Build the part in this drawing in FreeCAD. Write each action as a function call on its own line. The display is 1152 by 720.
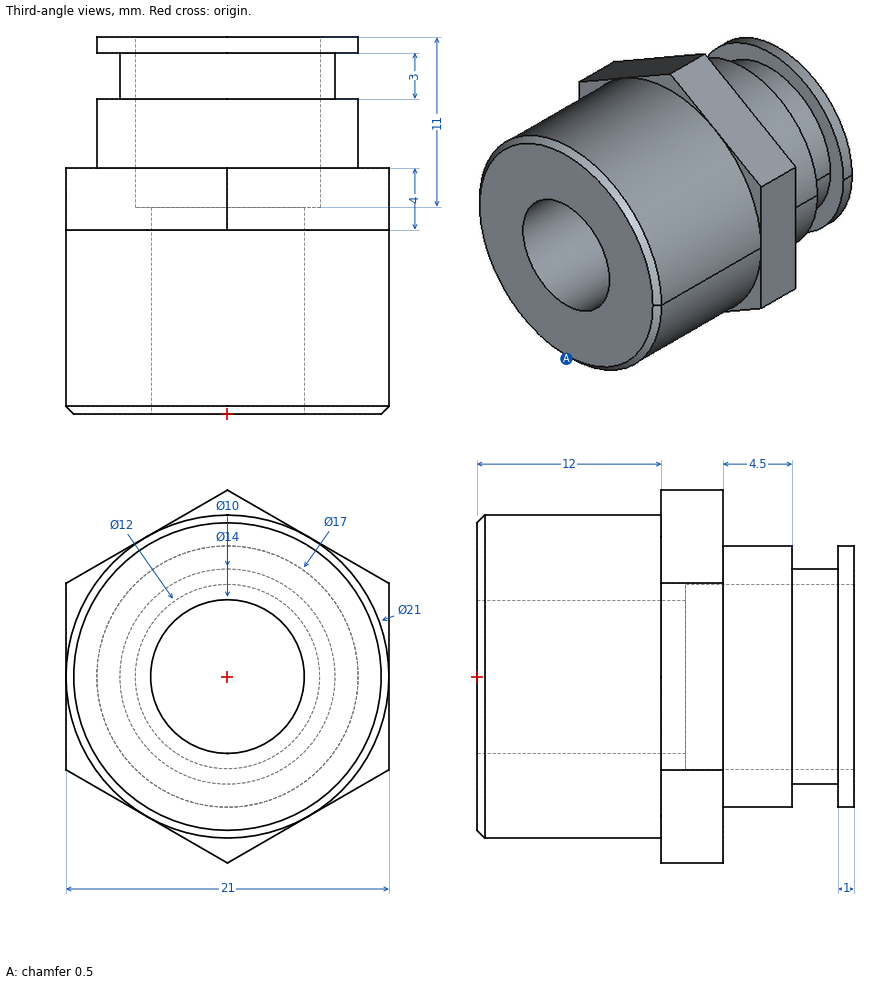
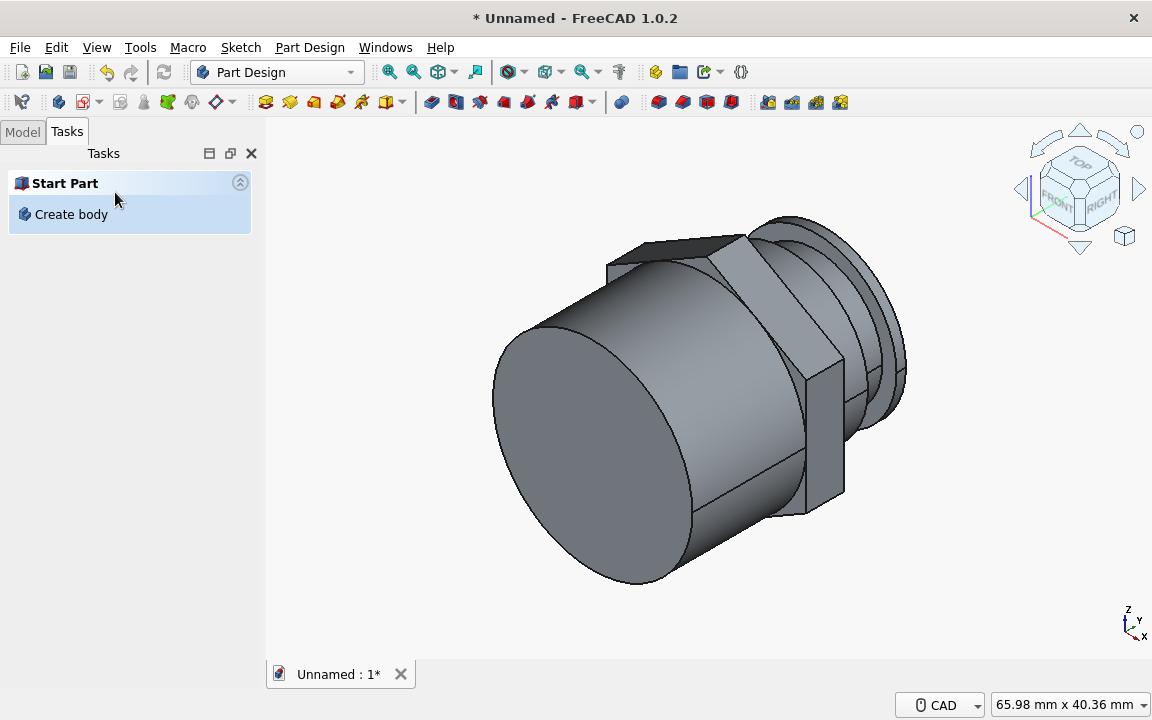
click(512, 340)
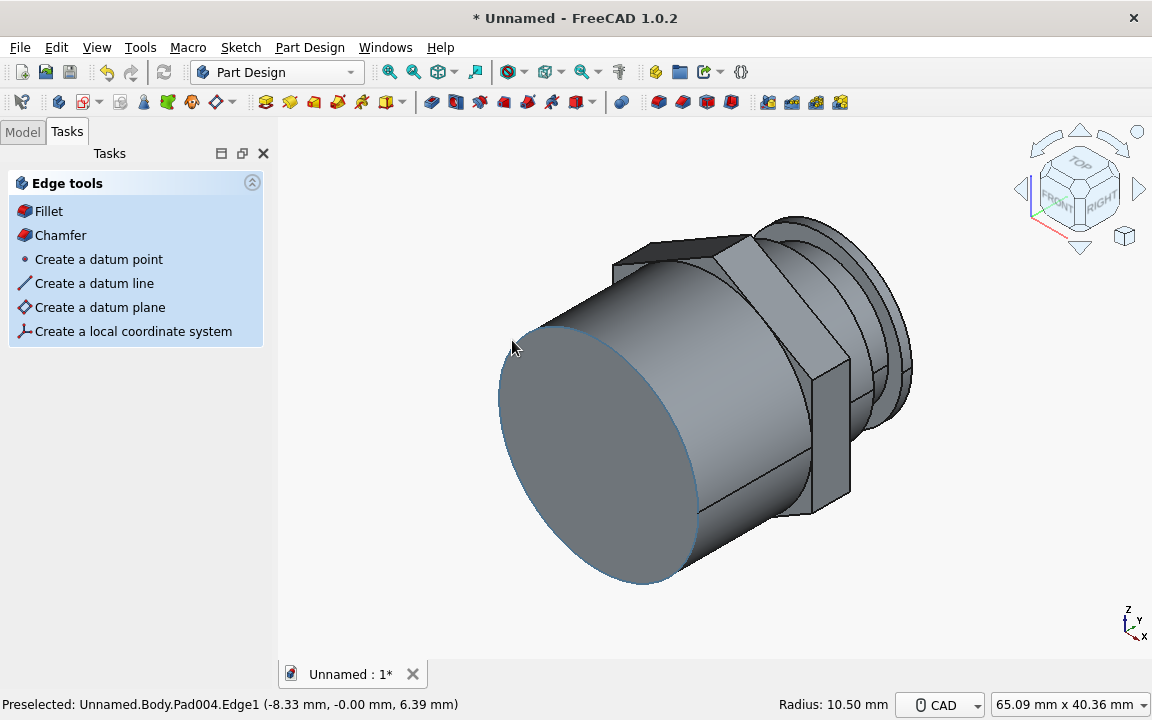
click(684, 102)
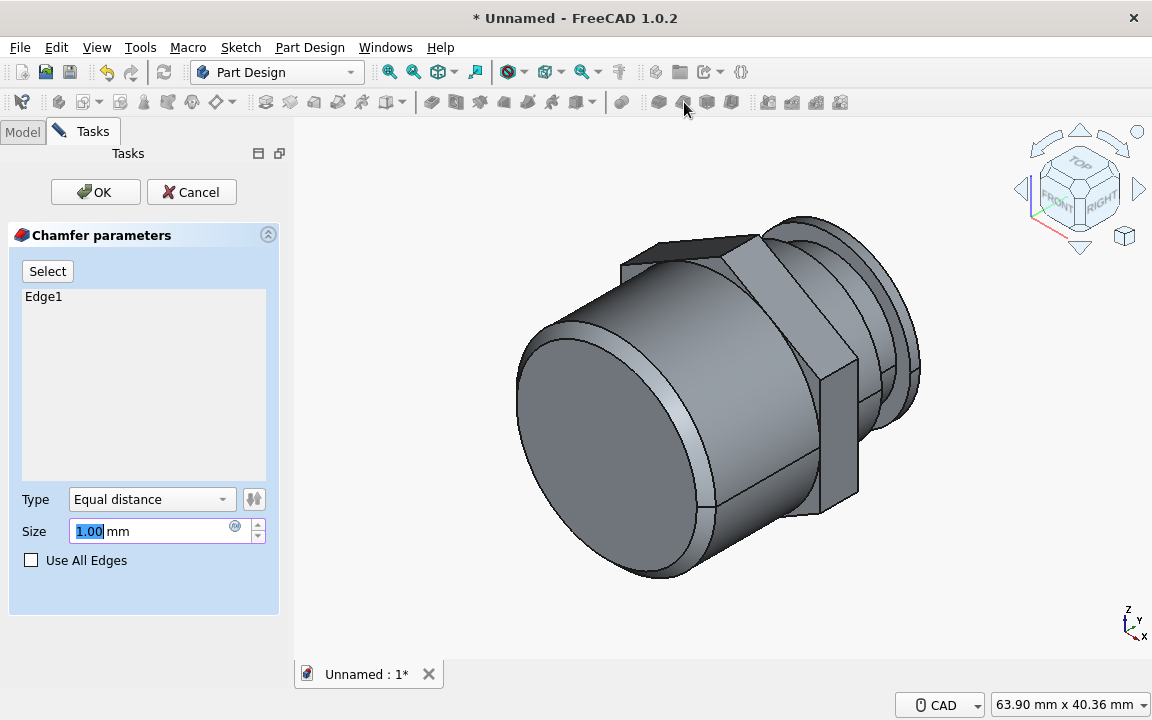
text(0.5)
key(Tab)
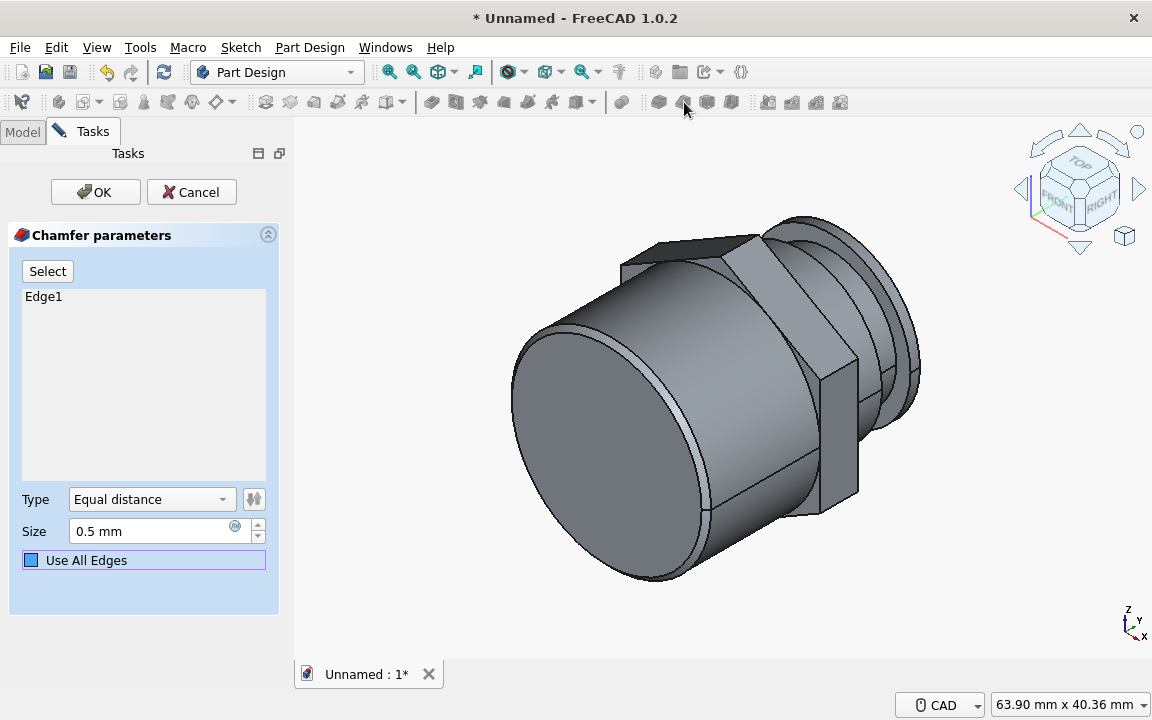
click(96, 192)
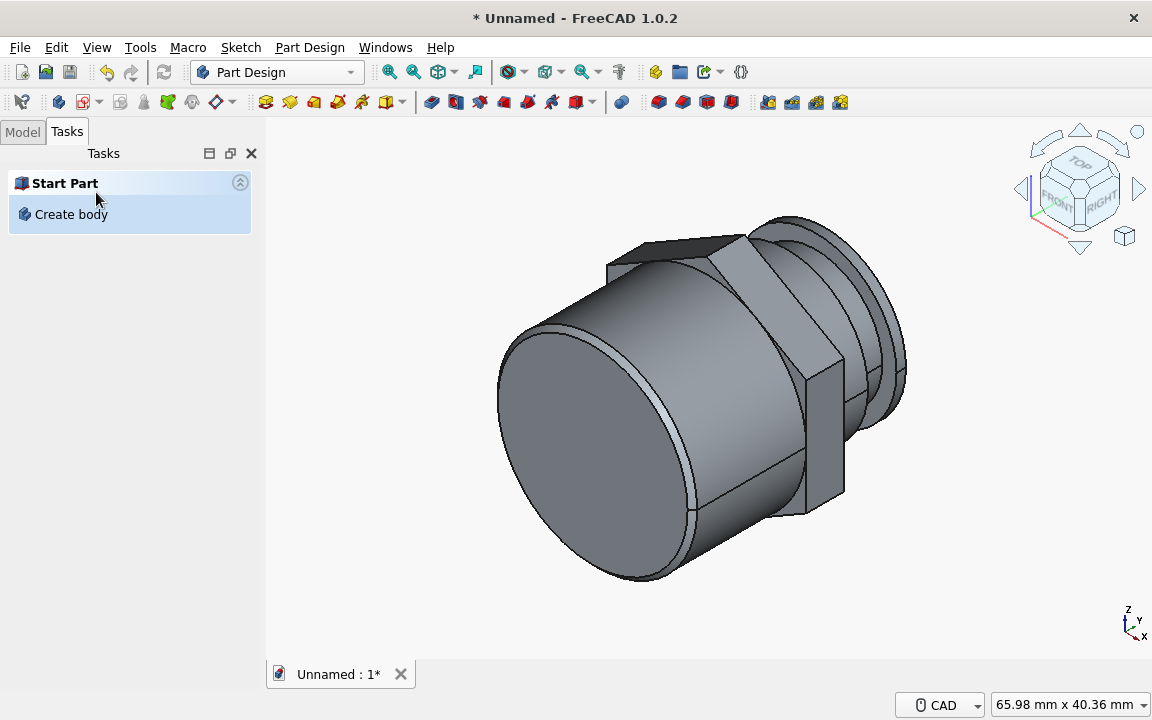
key(4)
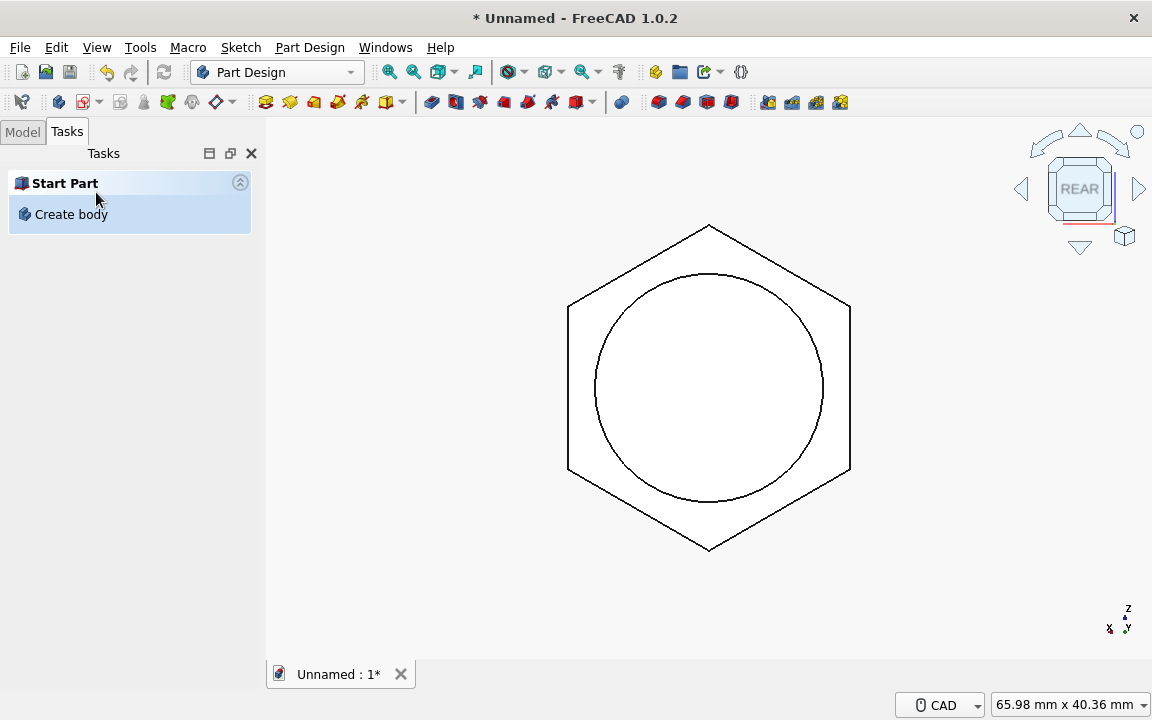
click(709, 387)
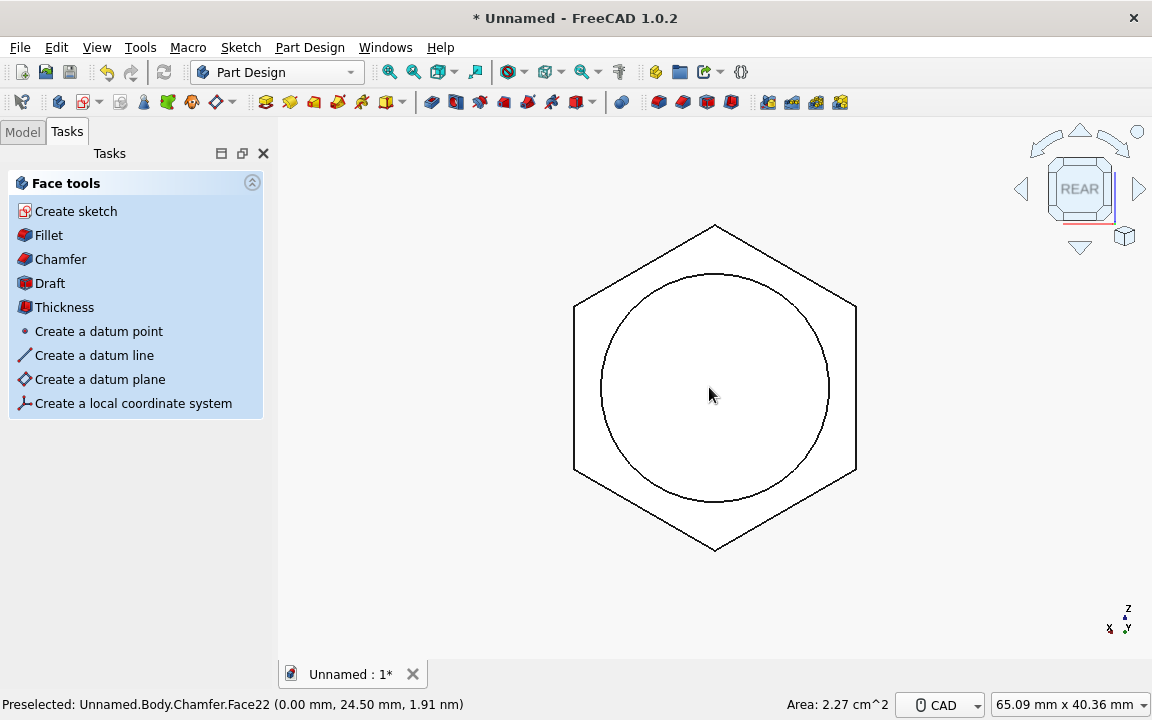
click(84, 102)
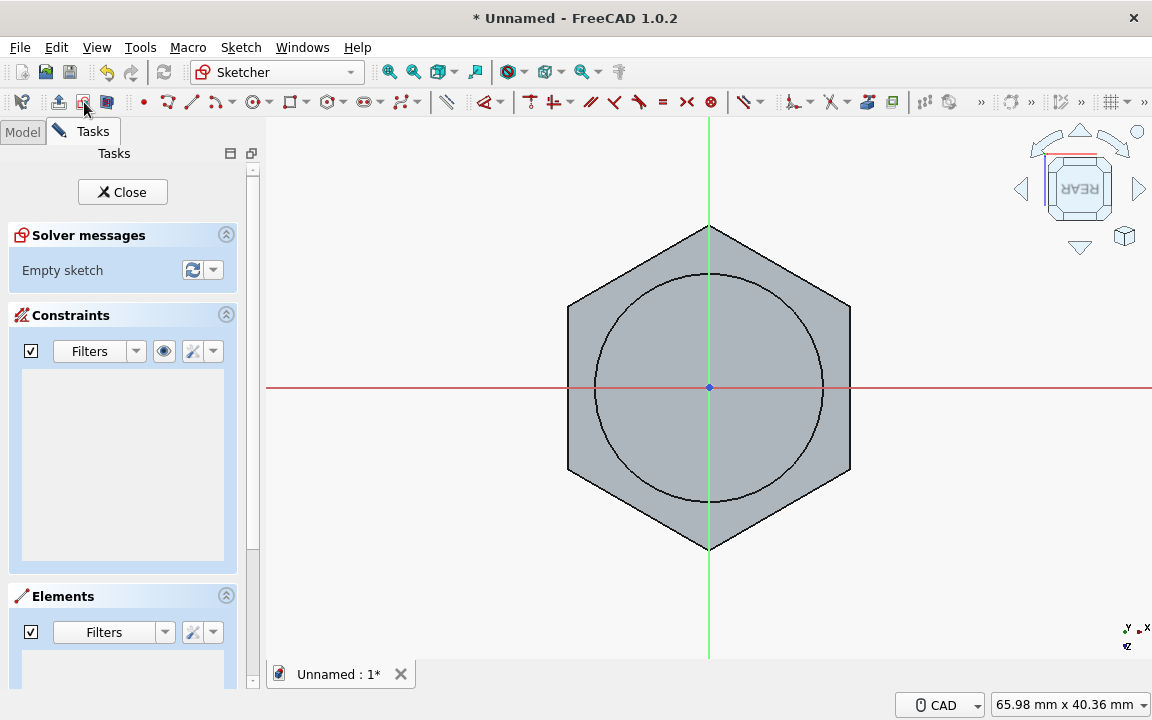
scroll(765, 388, up, 4)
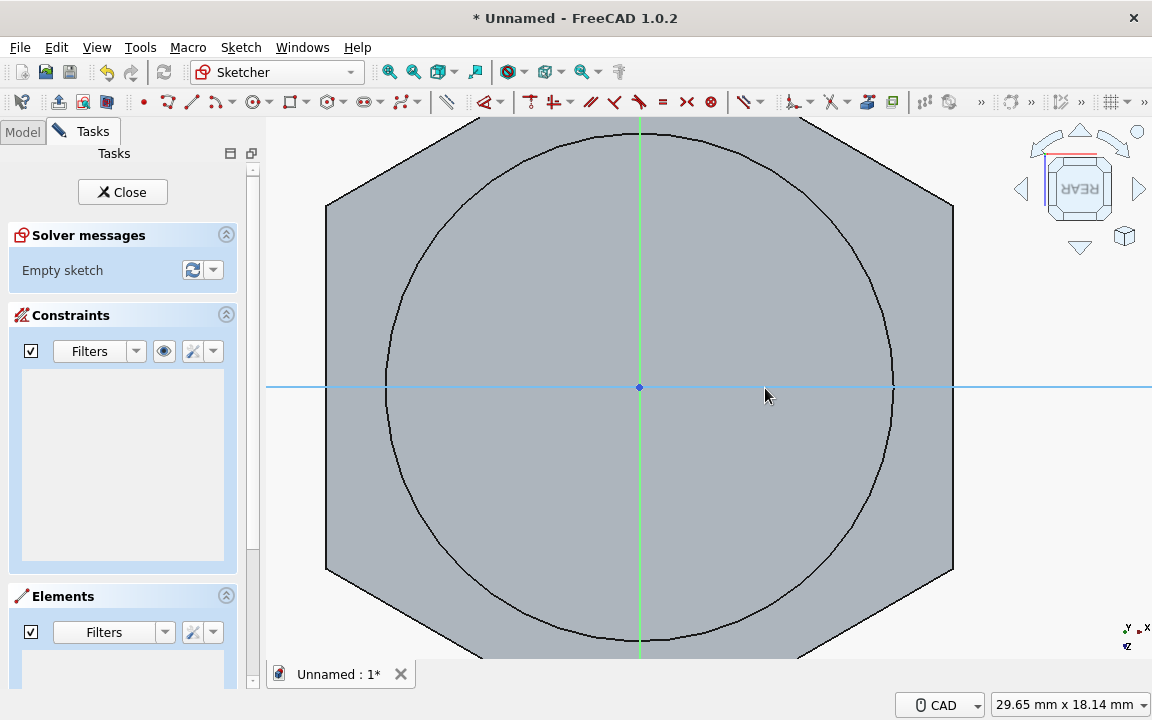
key(g)
key(c)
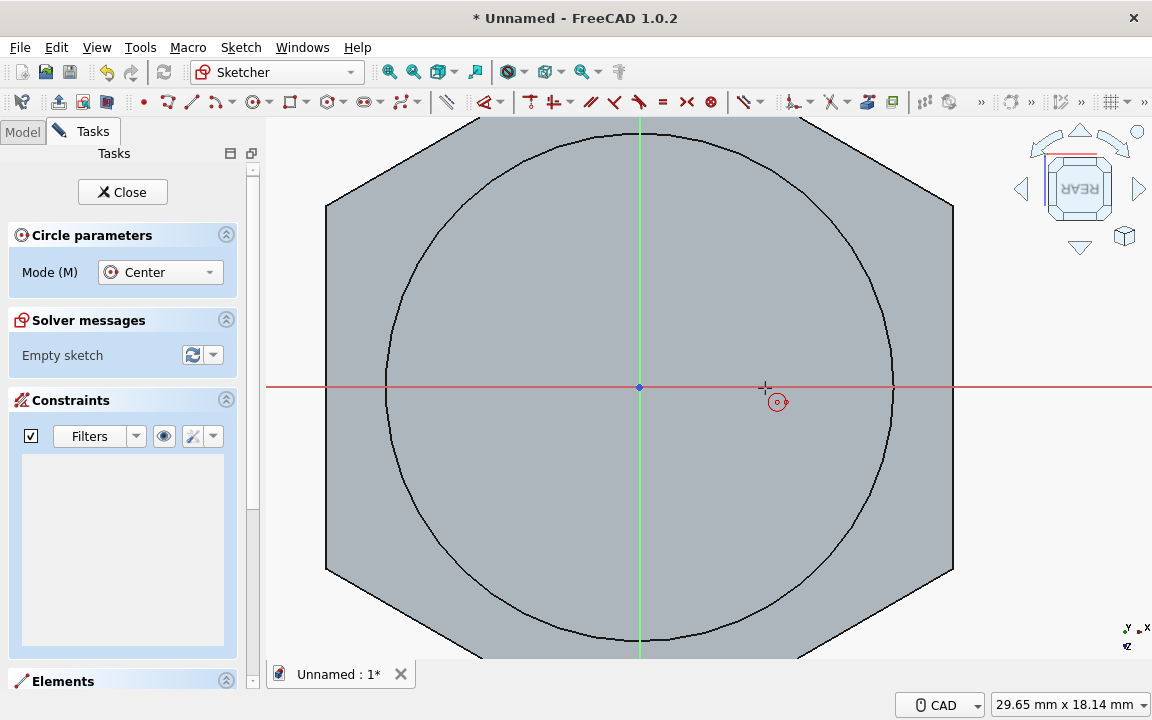
click(640, 387)
move(766, 261)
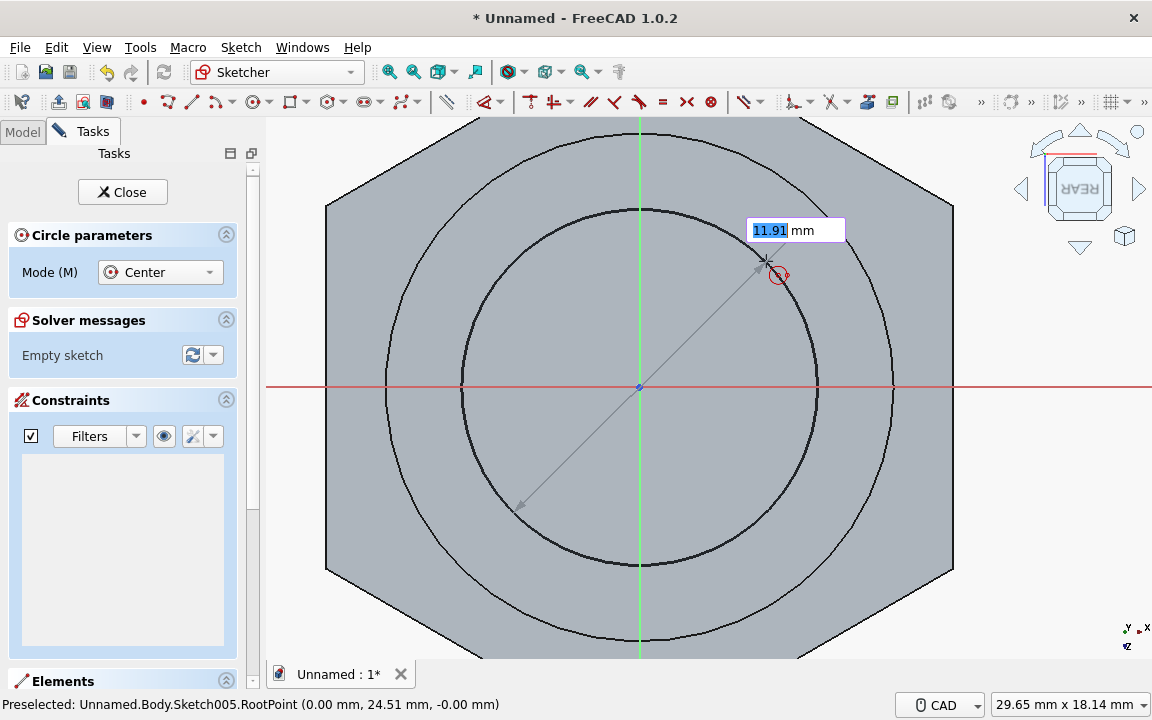
text(12)
key(Return)
key(Escape)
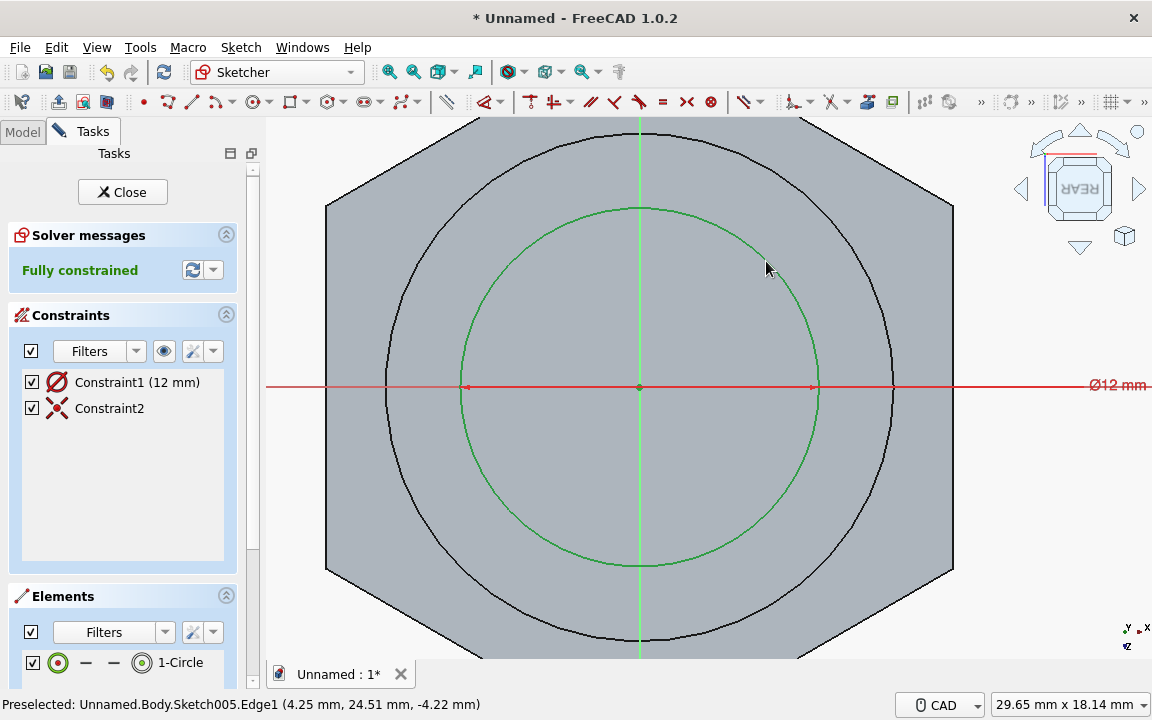
click(123, 192)